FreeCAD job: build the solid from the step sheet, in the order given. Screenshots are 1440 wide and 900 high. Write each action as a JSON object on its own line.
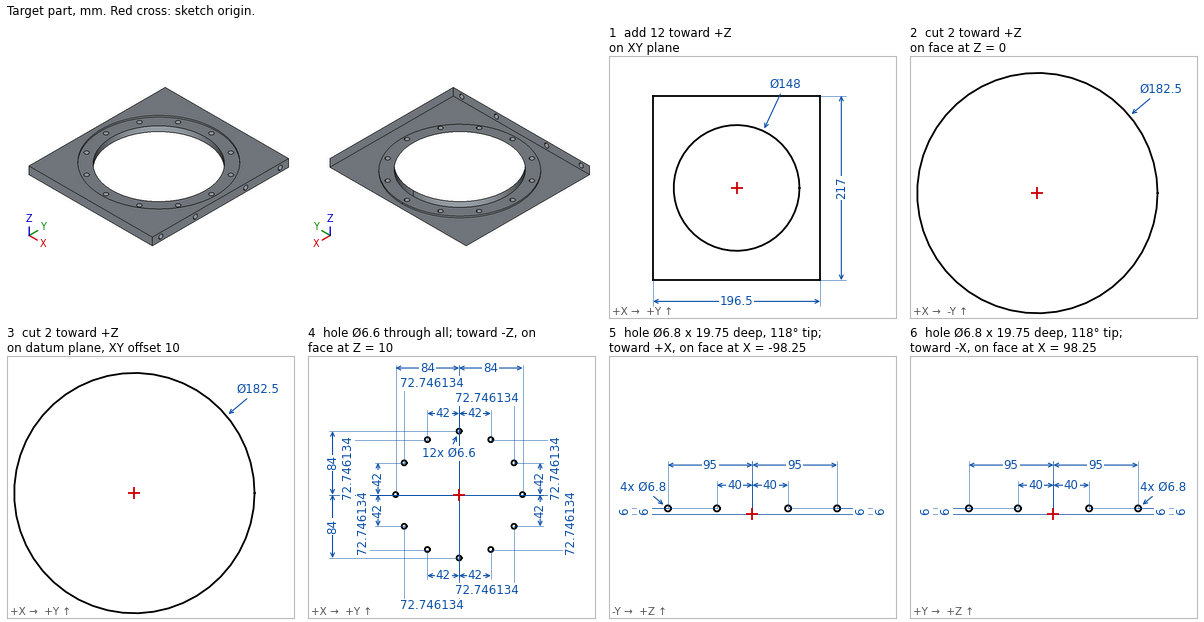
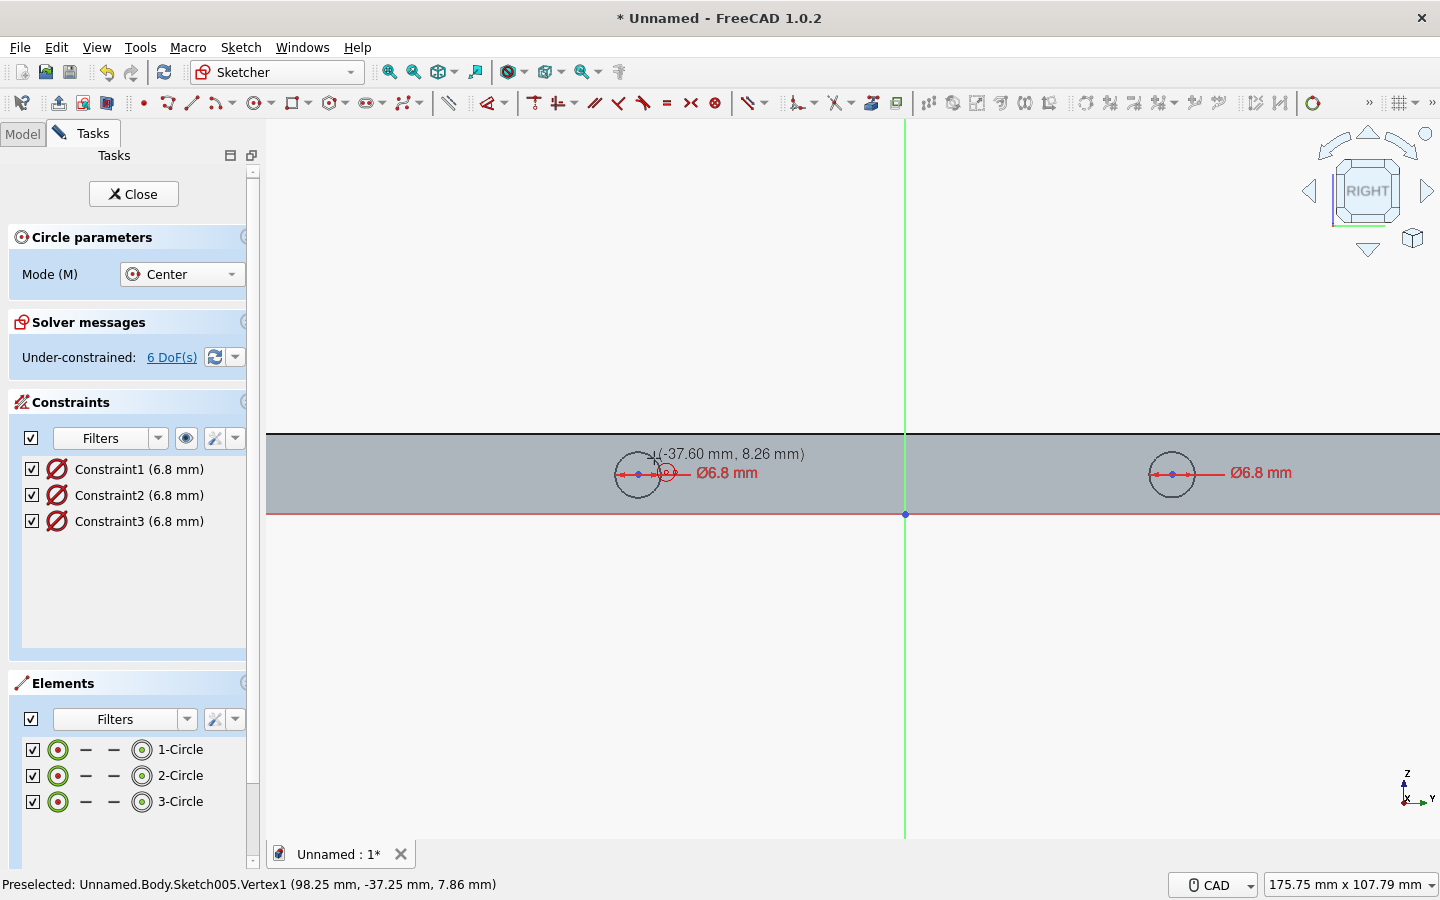
{"action": "scroll", "coordinate": [638, 474], "scroll_direction": "down", "scroll_amount": 3}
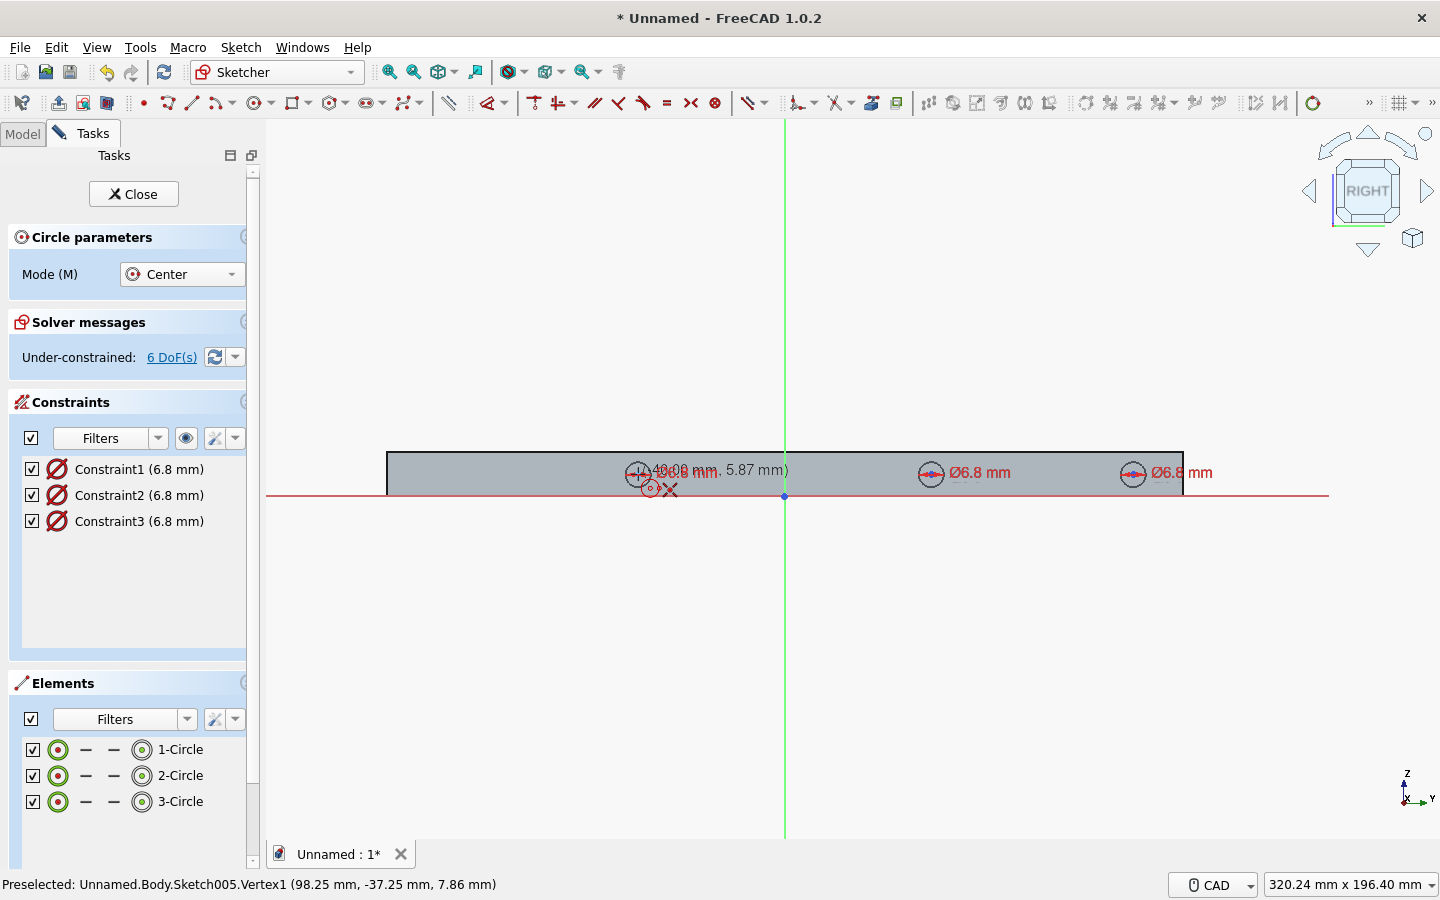
{"action": "scroll", "coordinate": [437, 474], "scroll_direction": "up", "scroll_amount": 3}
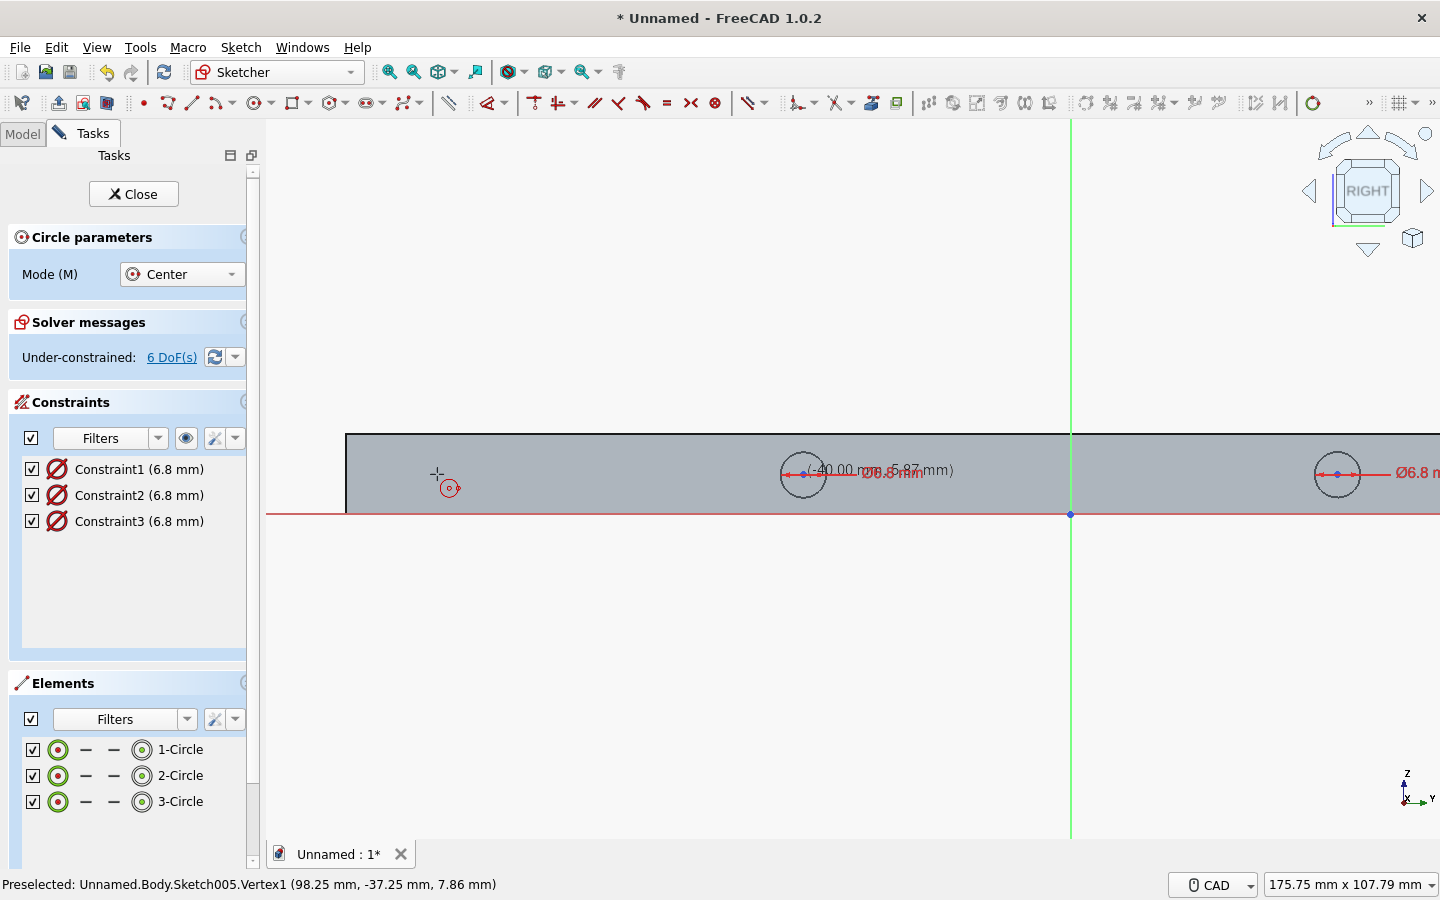
{"action": "left_click", "coordinate": [436, 474]}
{"action": "mouse_move", "coordinate": [452, 458]}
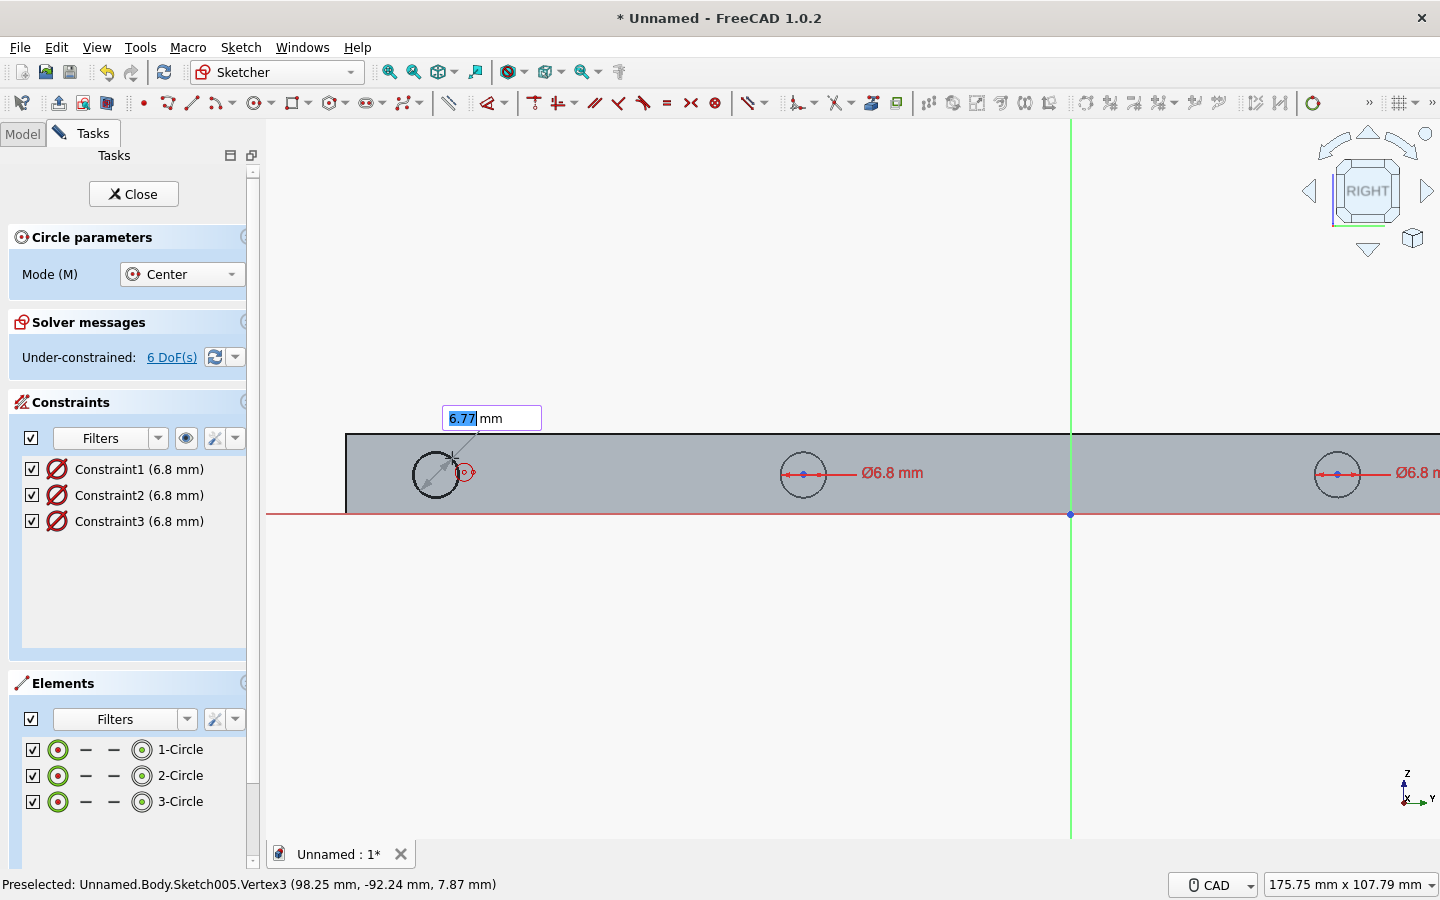
{"action": "type", "text": "6.8"}
{"action": "key", "text": "Return"}
{"action": "key", "text": "Escape"}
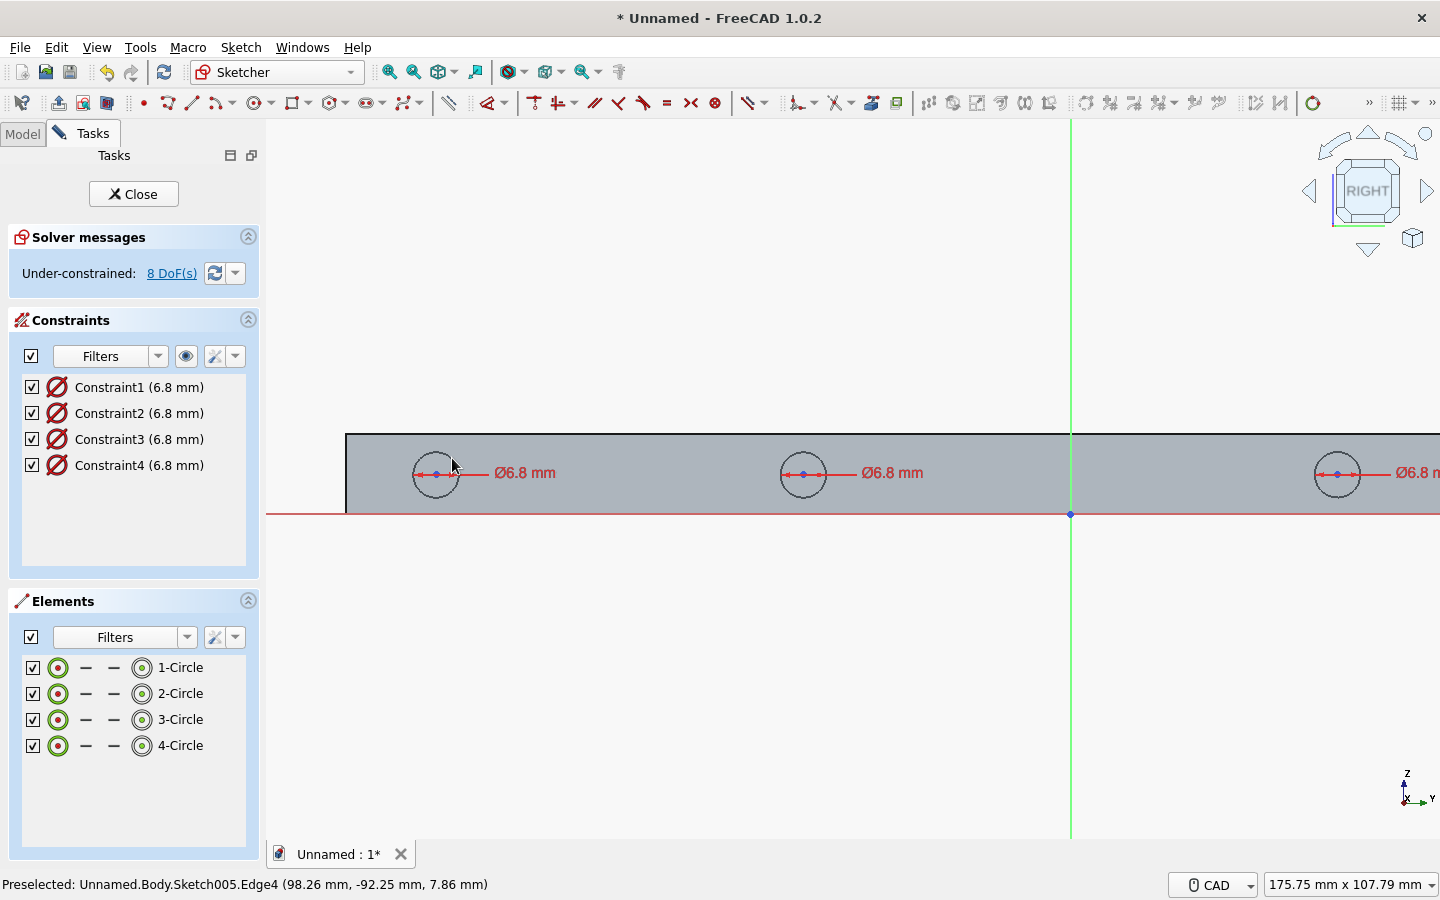
{"action": "left_click", "coordinate": [488, 104]}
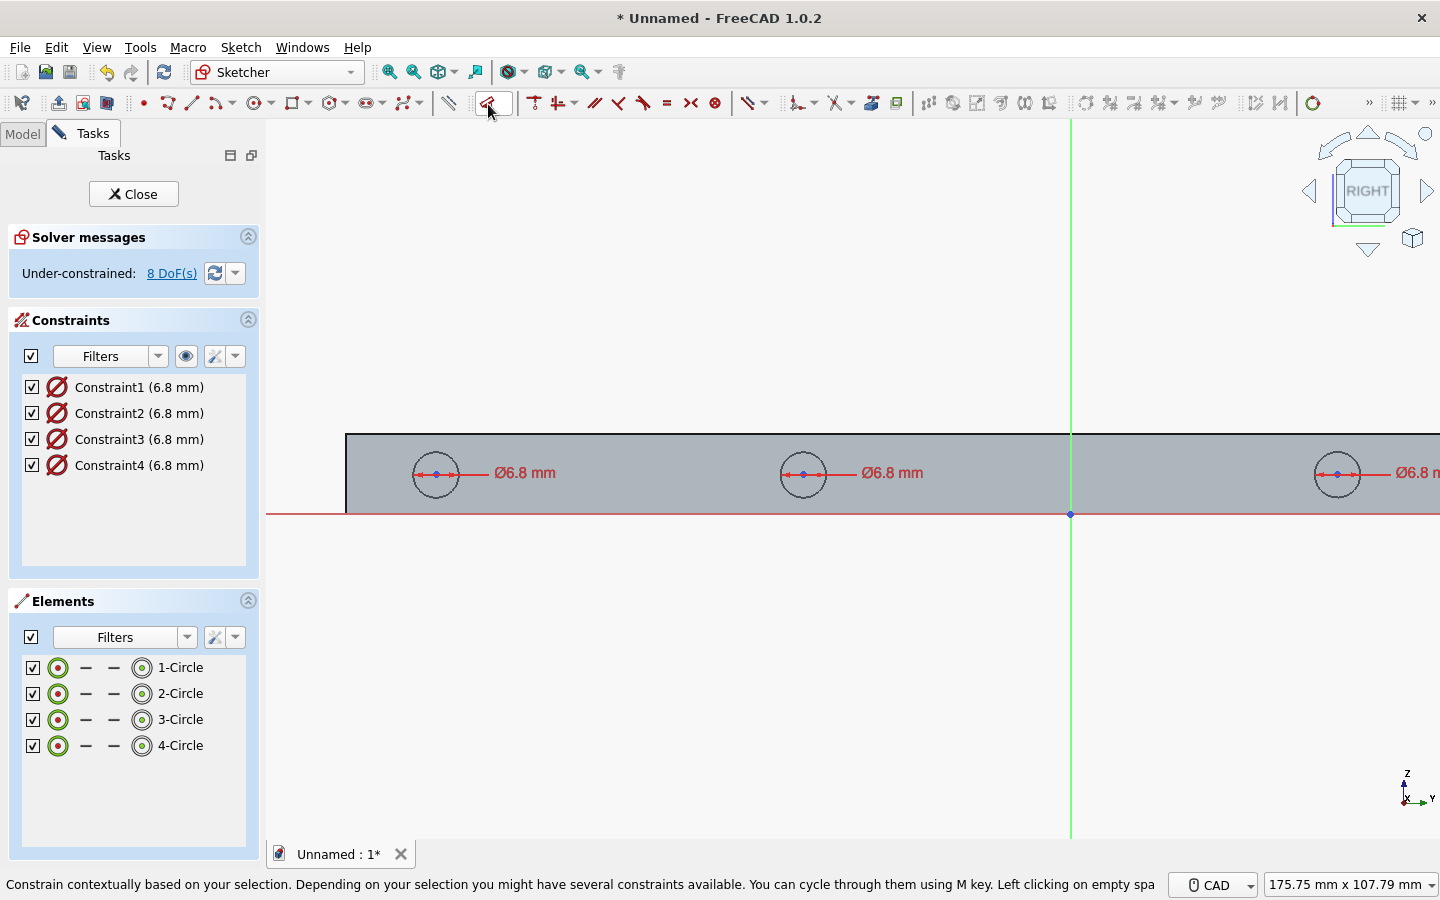
{"action": "scroll", "coordinate": [437, 474], "scroll_direction": "down", "scroll_amount": 3}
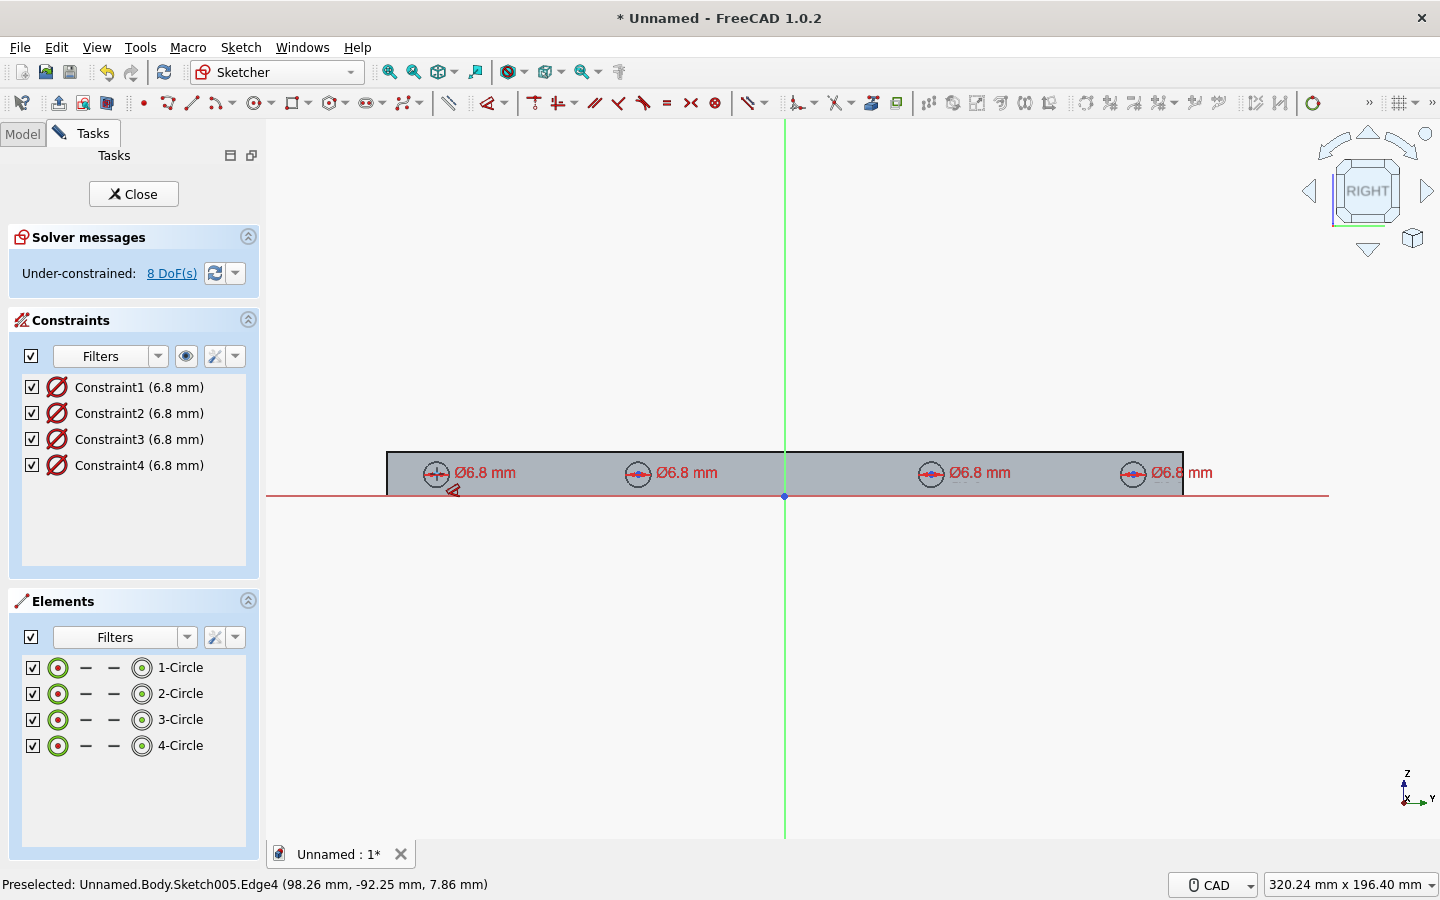
{"action": "scroll", "coordinate": [1133, 475], "scroll_direction": "up", "scroll_amount": 3}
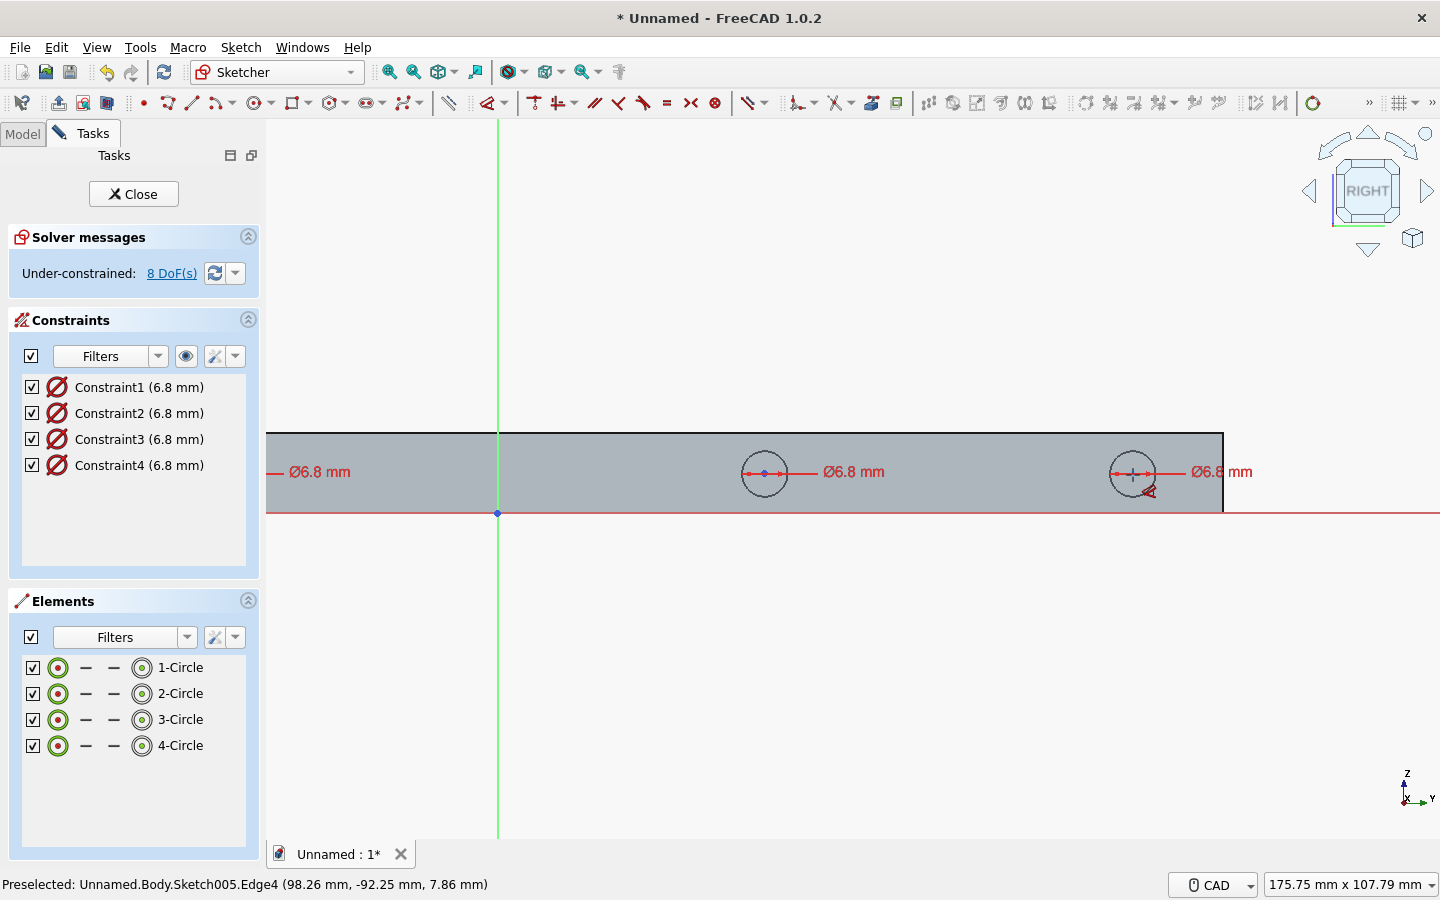
{"action": "left_click", "coordinate": [1133, 474]}
{"action": "left_click", "coordinate": [1167, 494]}